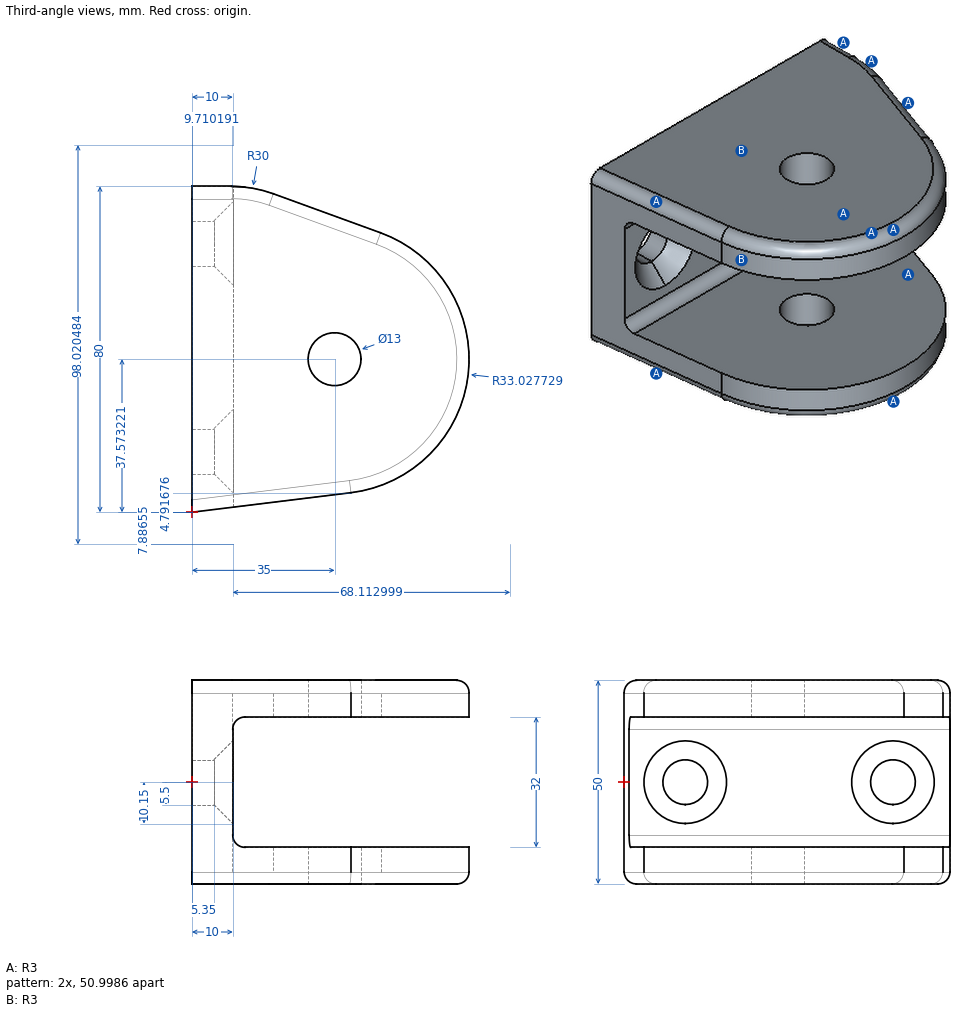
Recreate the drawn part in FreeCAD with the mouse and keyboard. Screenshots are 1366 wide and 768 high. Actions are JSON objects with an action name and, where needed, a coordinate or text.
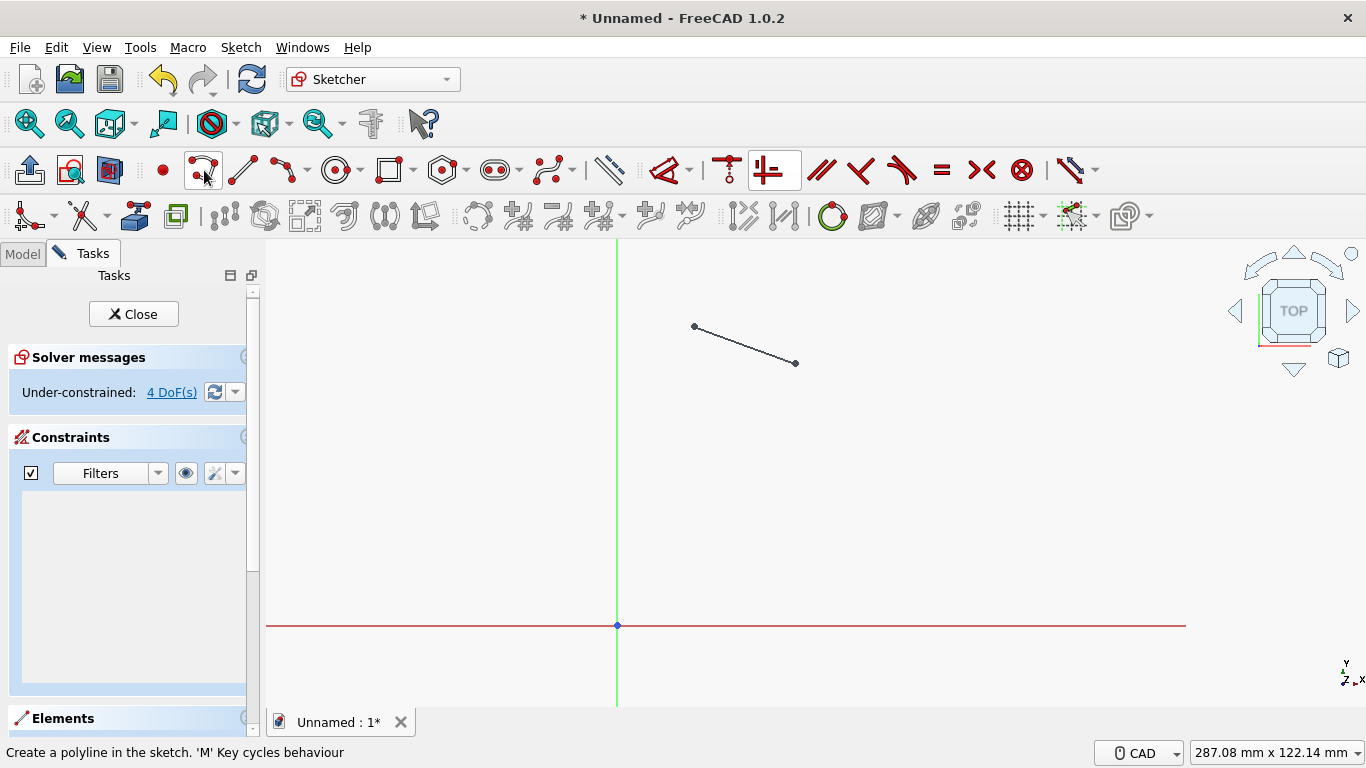
{"action": "left_click", "coordinate": [654, 319]}
{"action": "left_click", "coordinate": [617, 319]}
{"action": "left_click", "coordinate": [617, 626]}
{"action": "left_click", "coordinate": [767, 607]}
{"action": "right_click", "coordinate": [767, 607]}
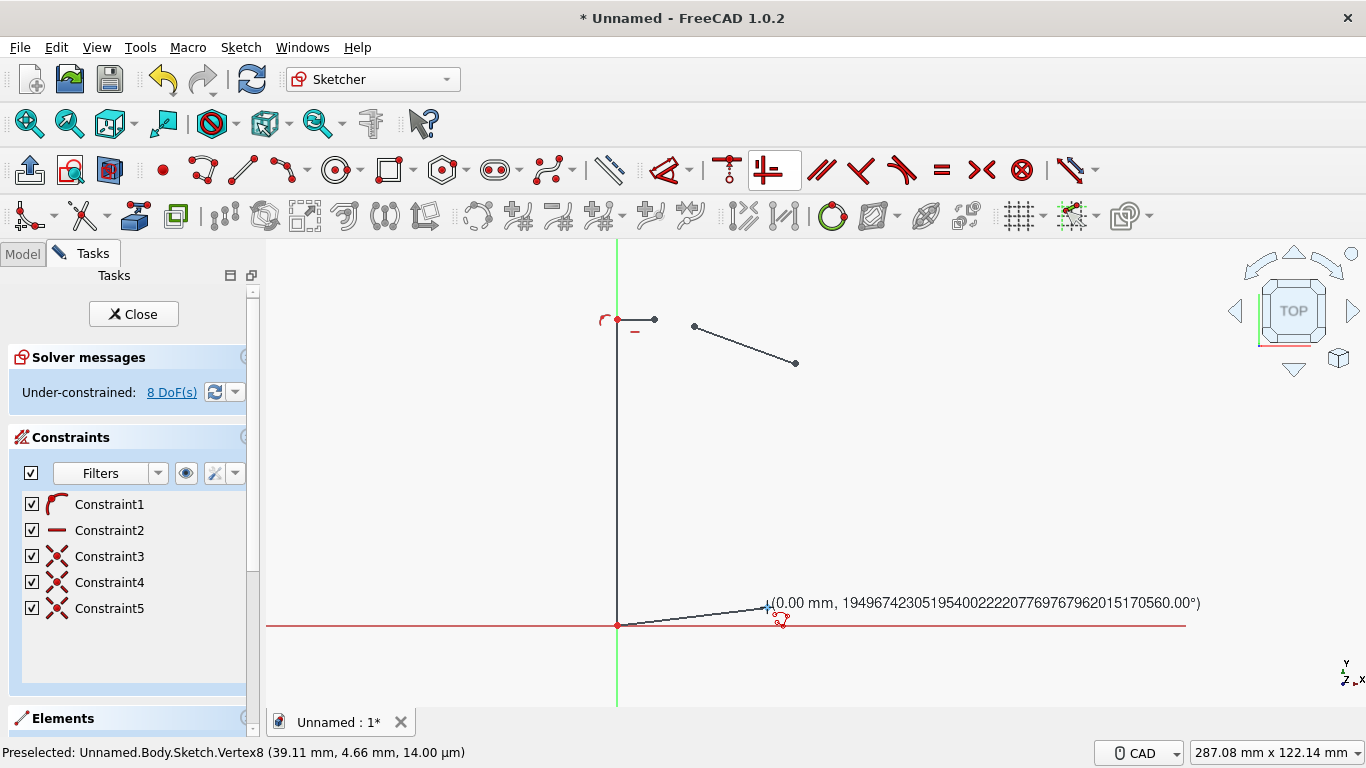
{"action": "left_click", "coordinate": [284, 170]}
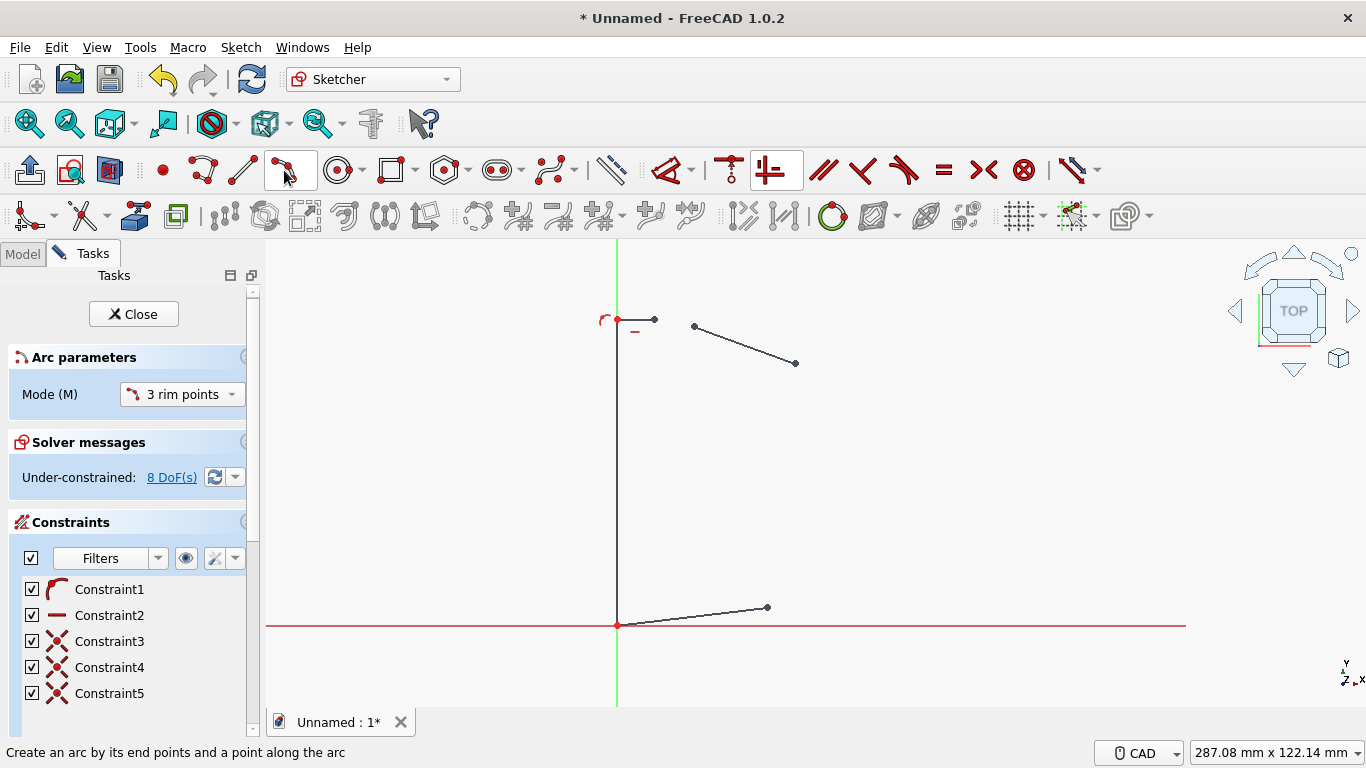
{"action": "left_click", "coordinate": [694, 327]}
{"action": "left_click", "coordinate": [654, 320]}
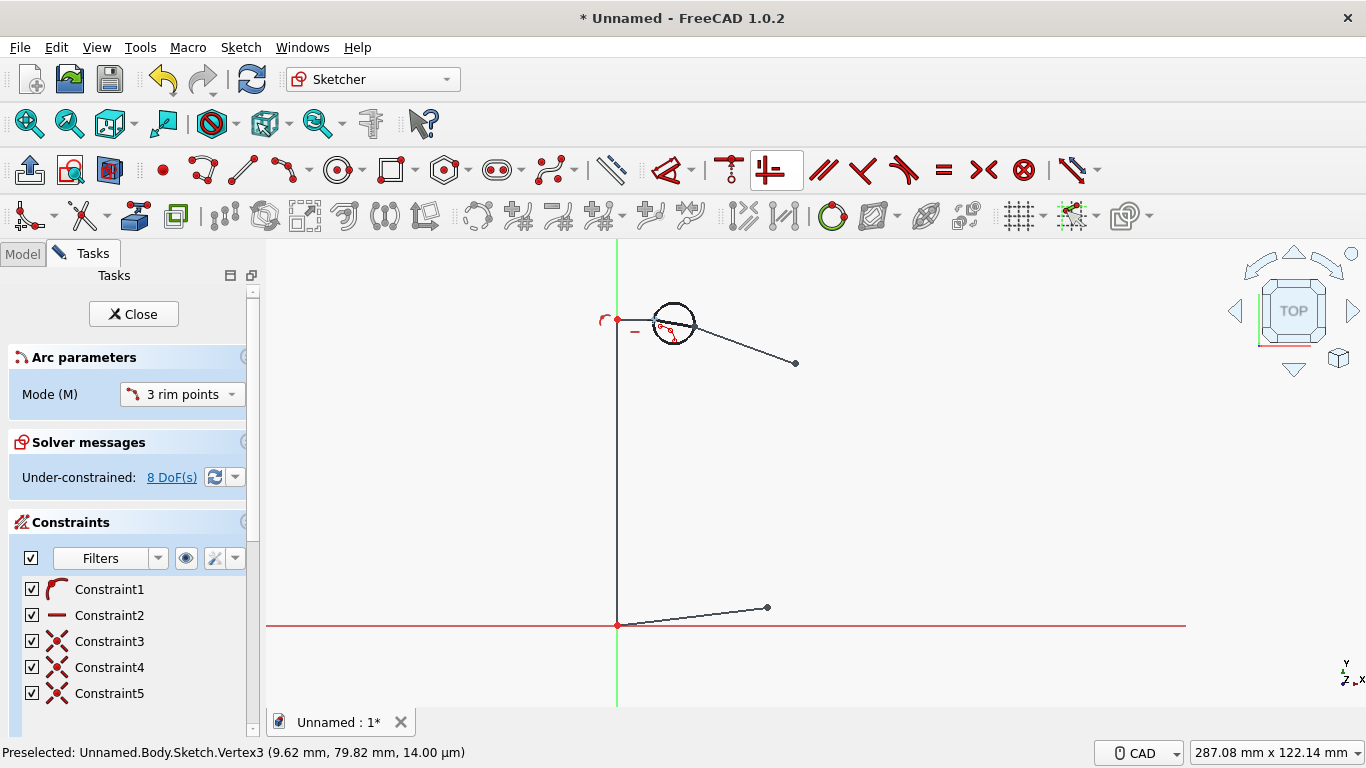
{"action": "scroll", "coordinate": [674, 321], "scroll_direction": "up", "scroll_amount": 12}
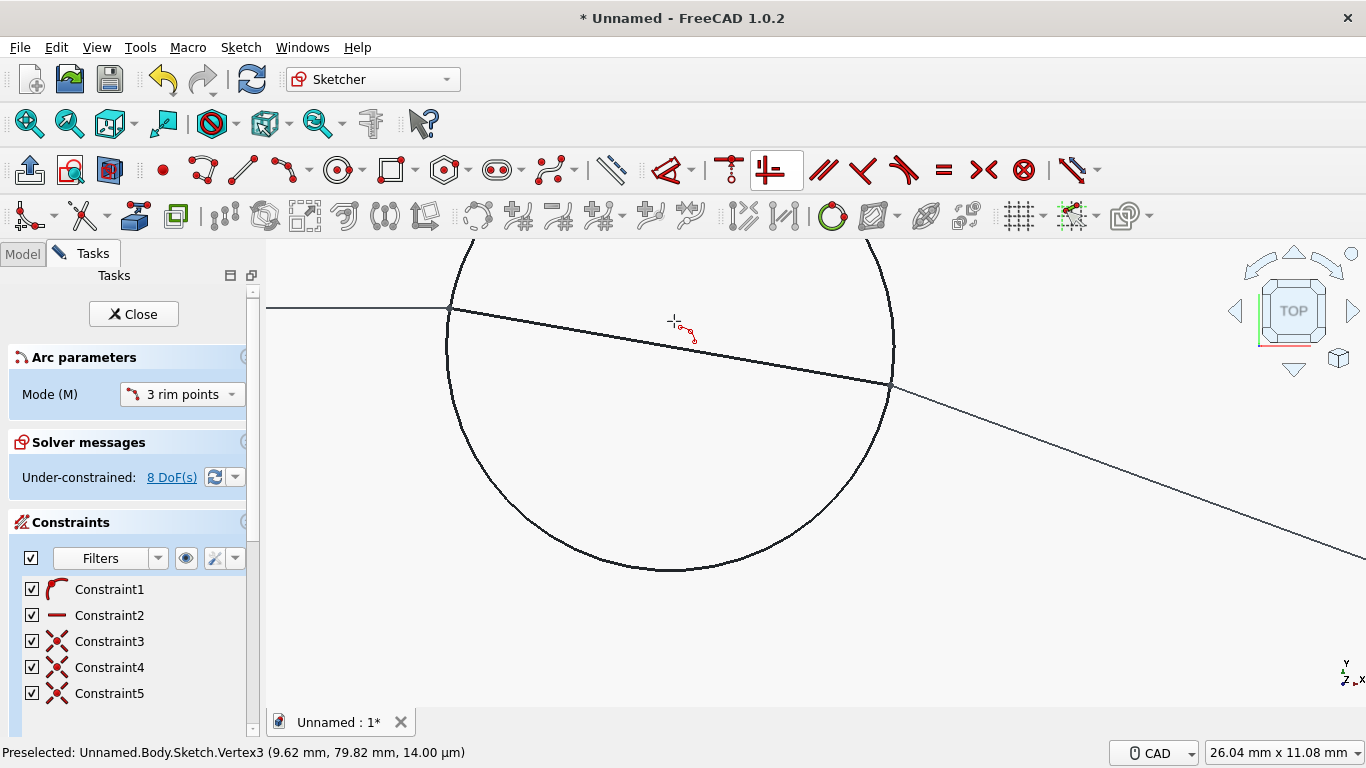
{"action": "left_click", "coordinate": [674, 320]}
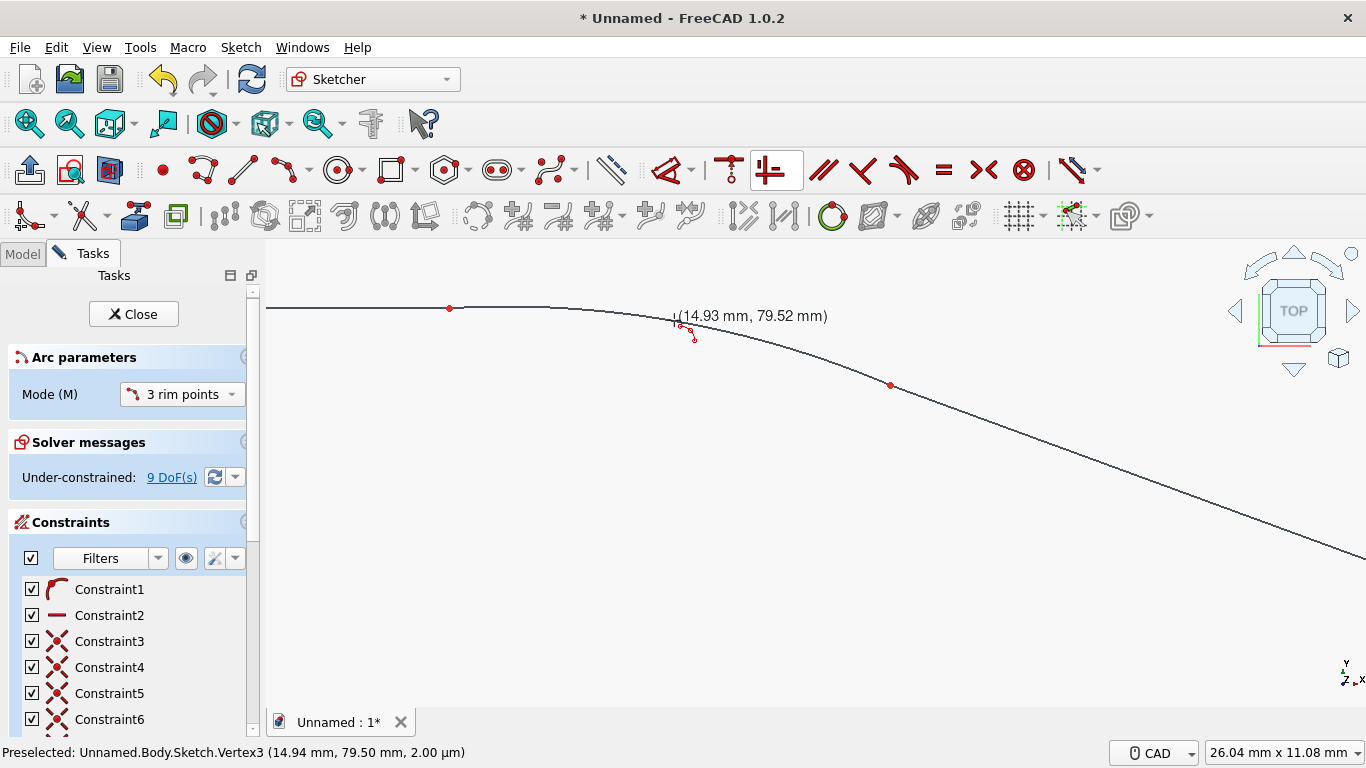
{"action": "scroll", "coordinate": [675, 322], "scroll_direction": "down", "scroll_amount": 12}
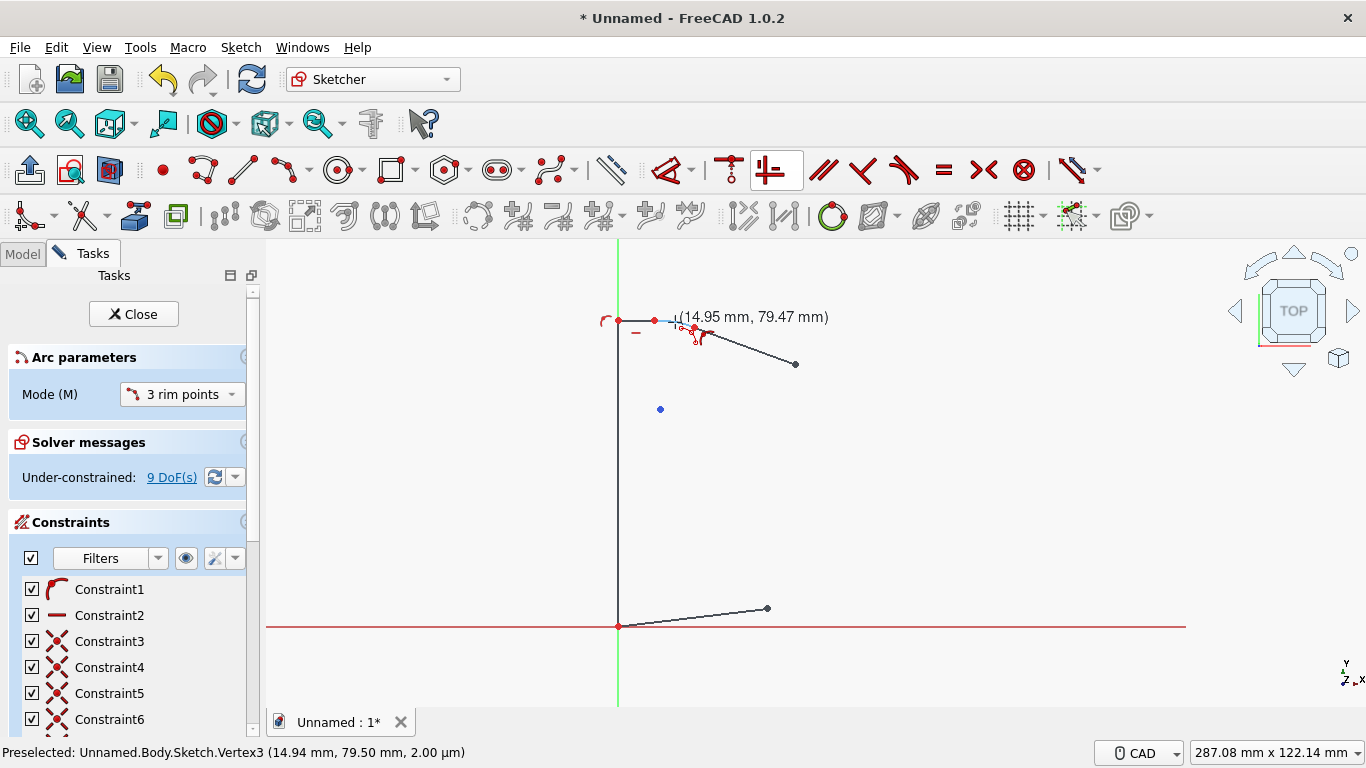
{"action": "left_click", "coordinate": [768, 609]}
{"action": "left_click", "coordinate": [796, 365]}
{"action": "left_click", "coordinate": [878, 497]}
{"action": "key", "text": "Escape"}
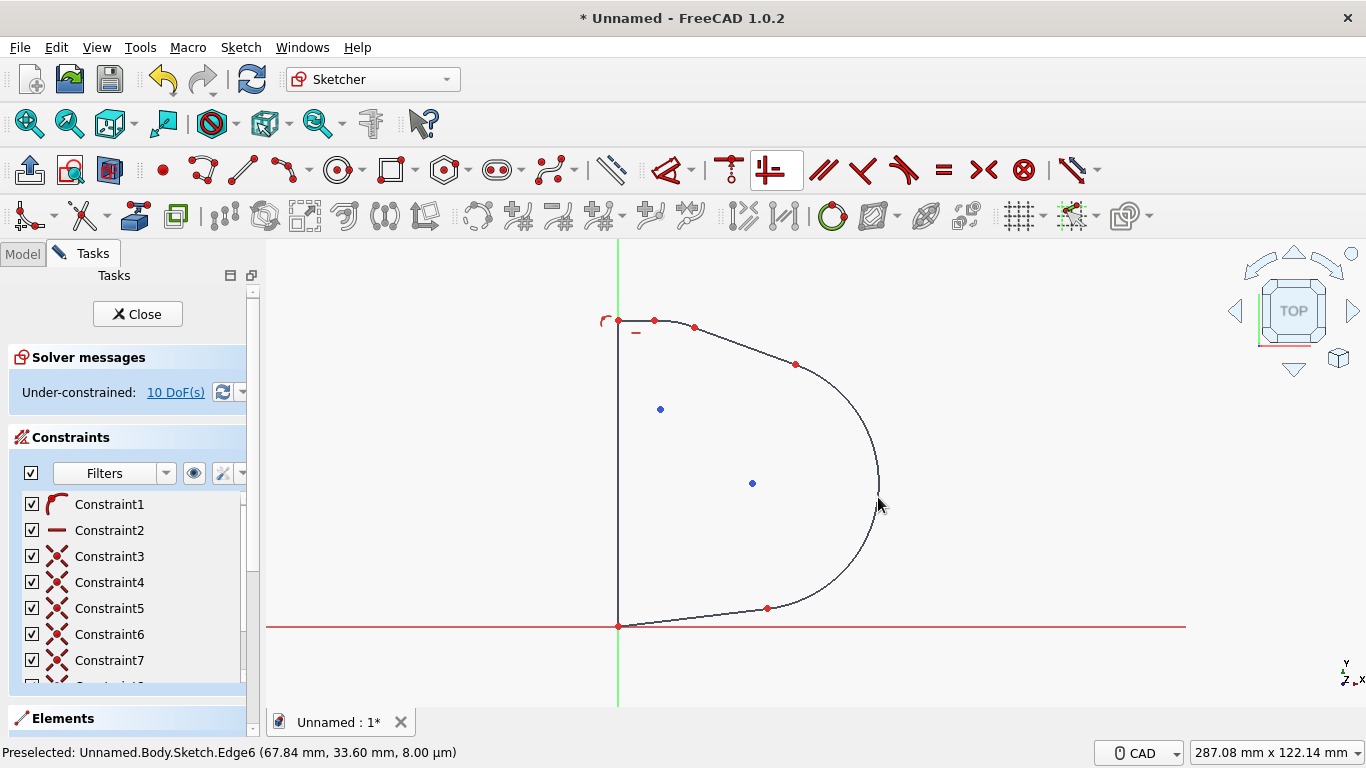
{"action": "left_click", "coordinate": [766, 354]}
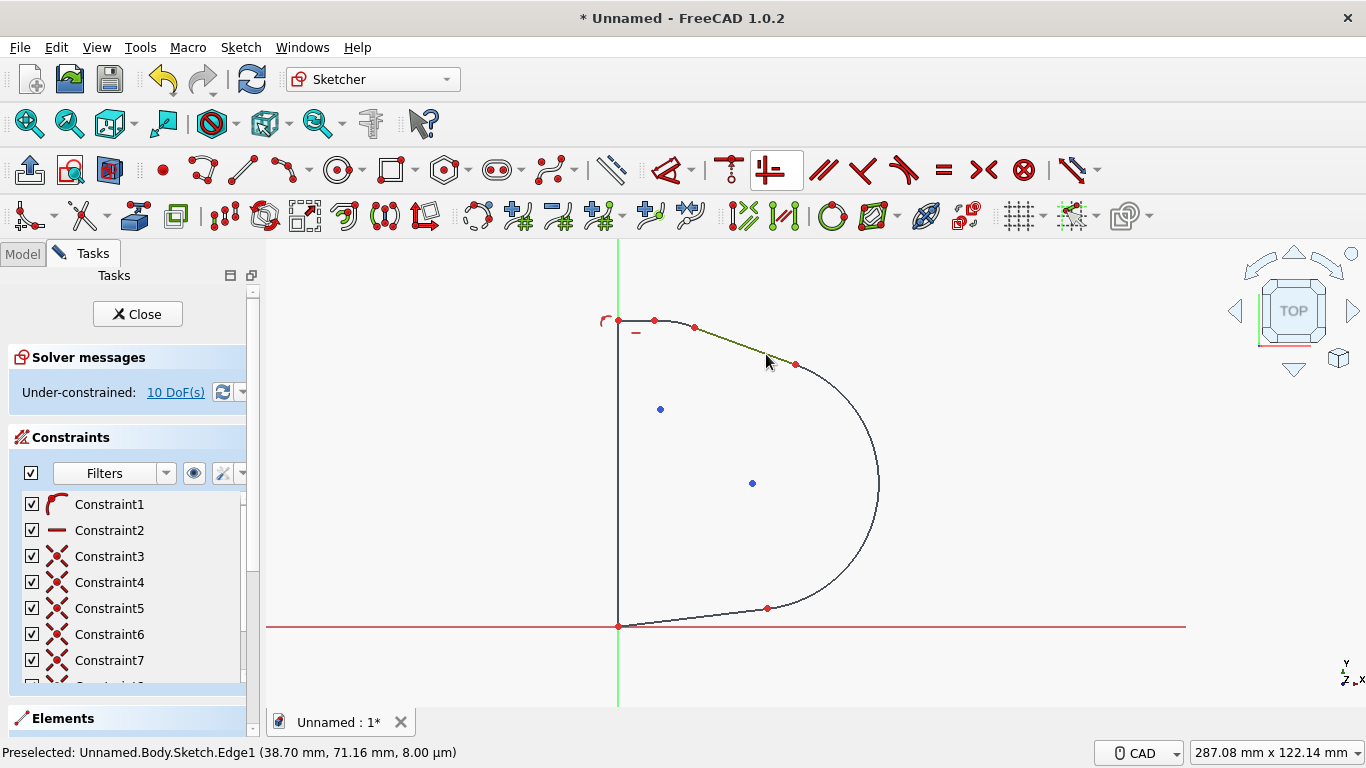
{"action": "left_click", "coordinate": [683, 324]}